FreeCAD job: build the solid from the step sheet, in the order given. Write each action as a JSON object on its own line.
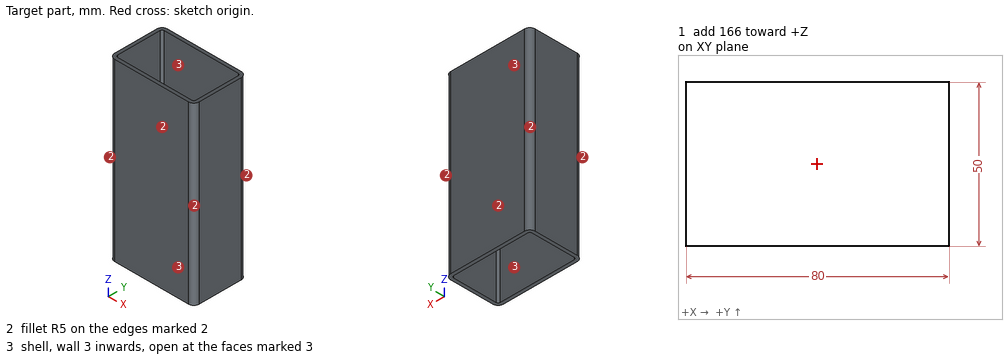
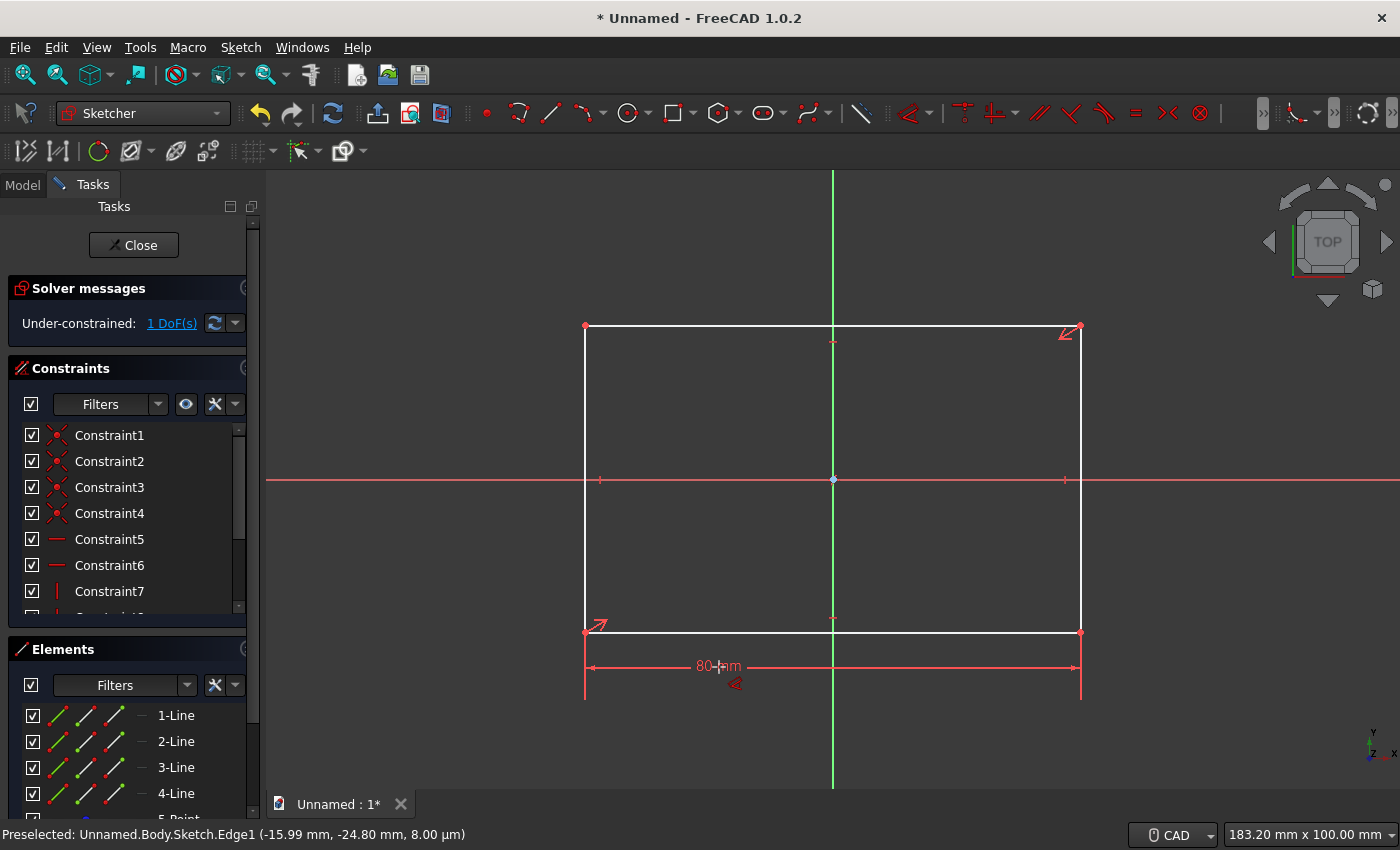
{"action": "left_click", "coordinate": [1081, 541]}
{"action": "left_click", "coordinate": [1115, 409]}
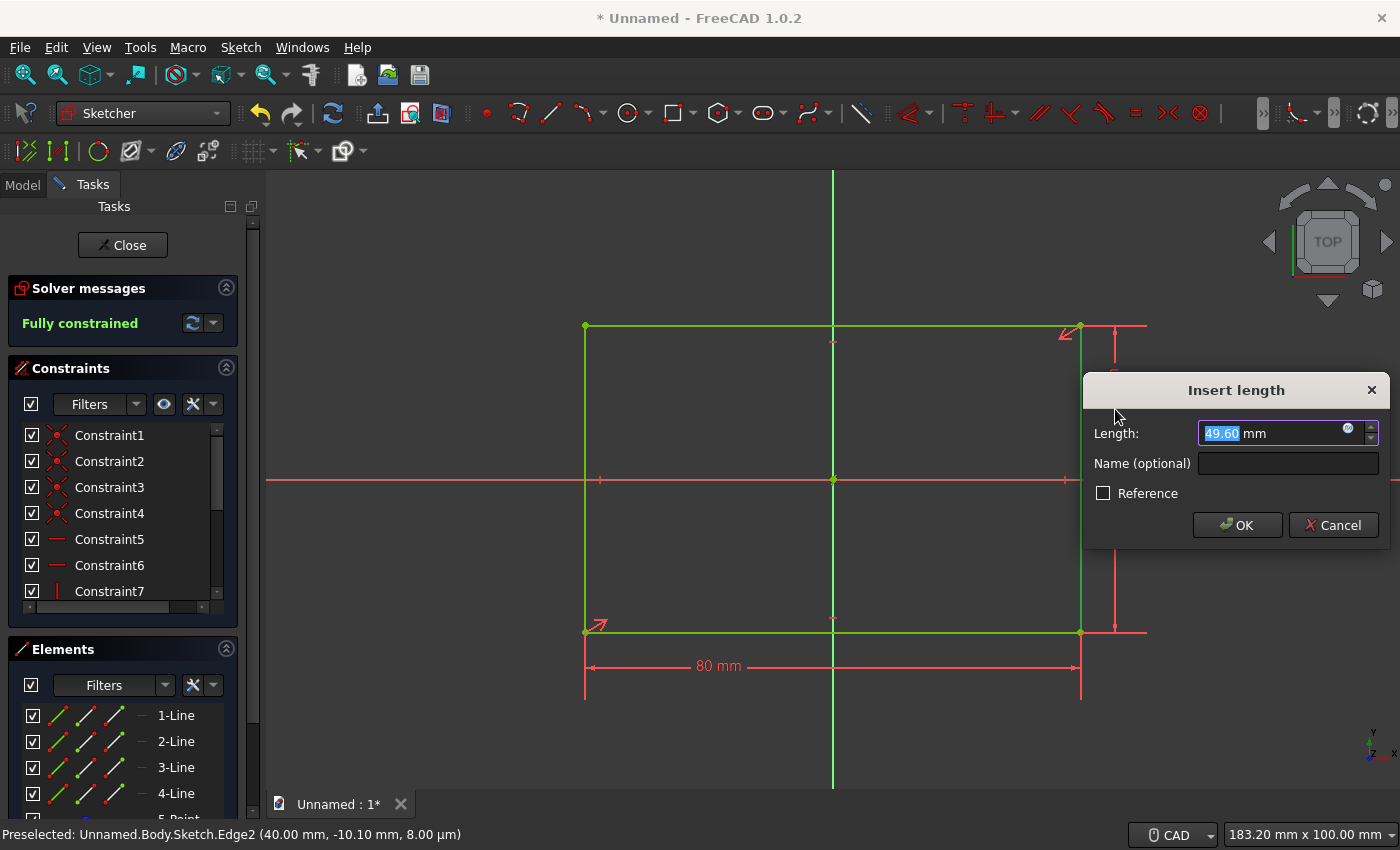
{"action": "type", "text": "50"}
{"action": "key", "text": "Return"}
{"action": "key", "text": "Escape"}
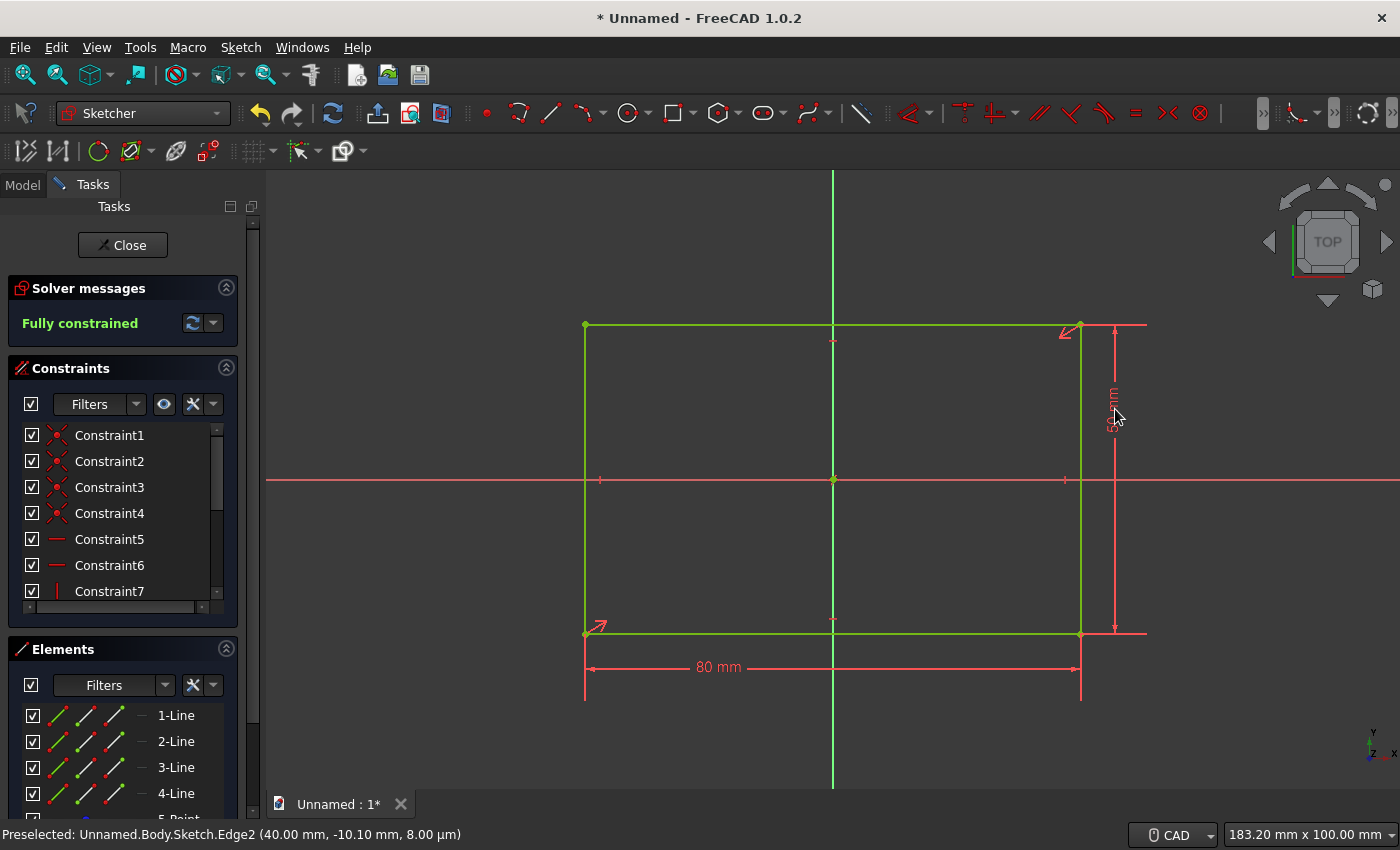
{"action": "left_click", "coordinate": [123, 245]}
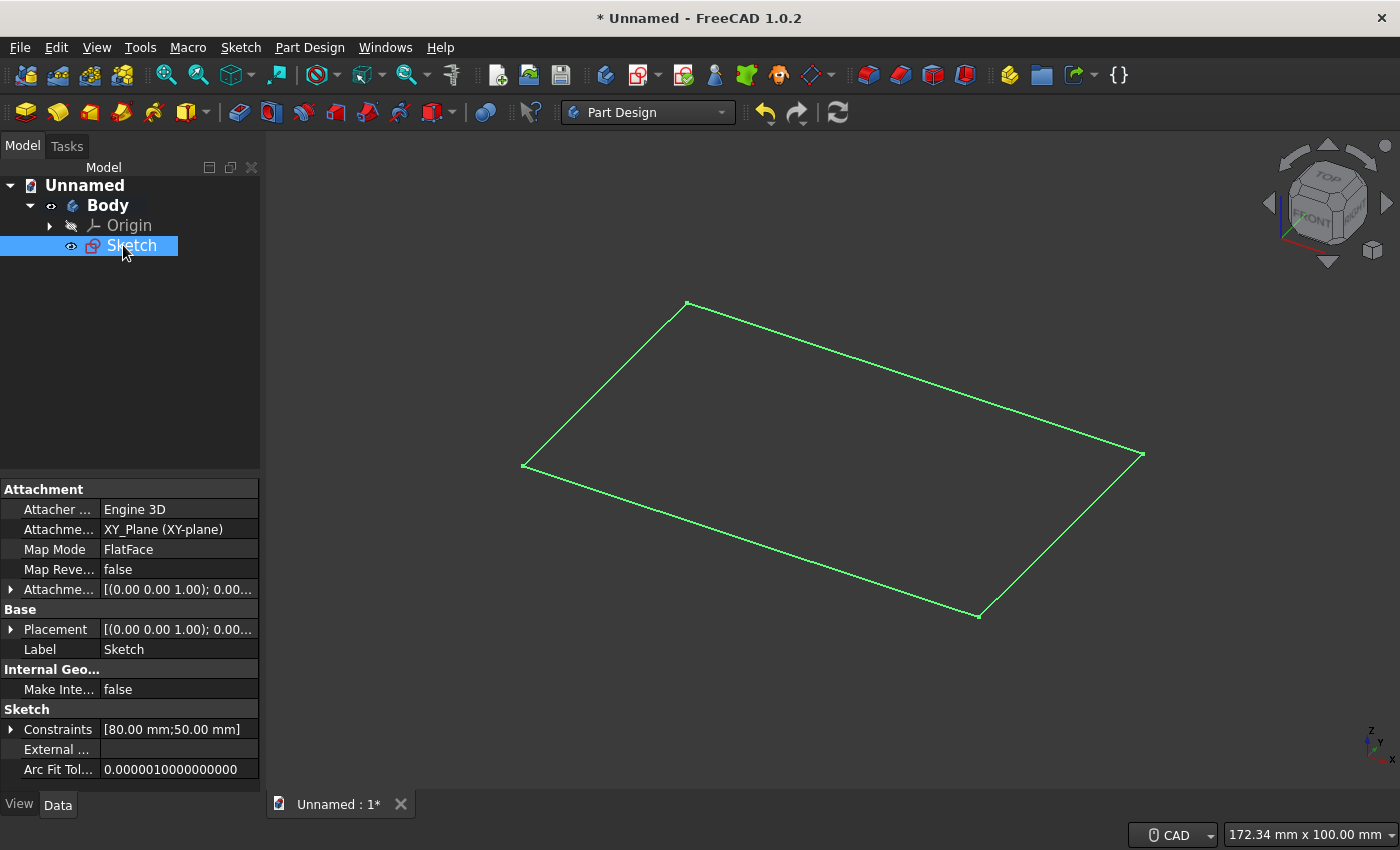
{"action": "left_click", "coordinate": [26, 112]}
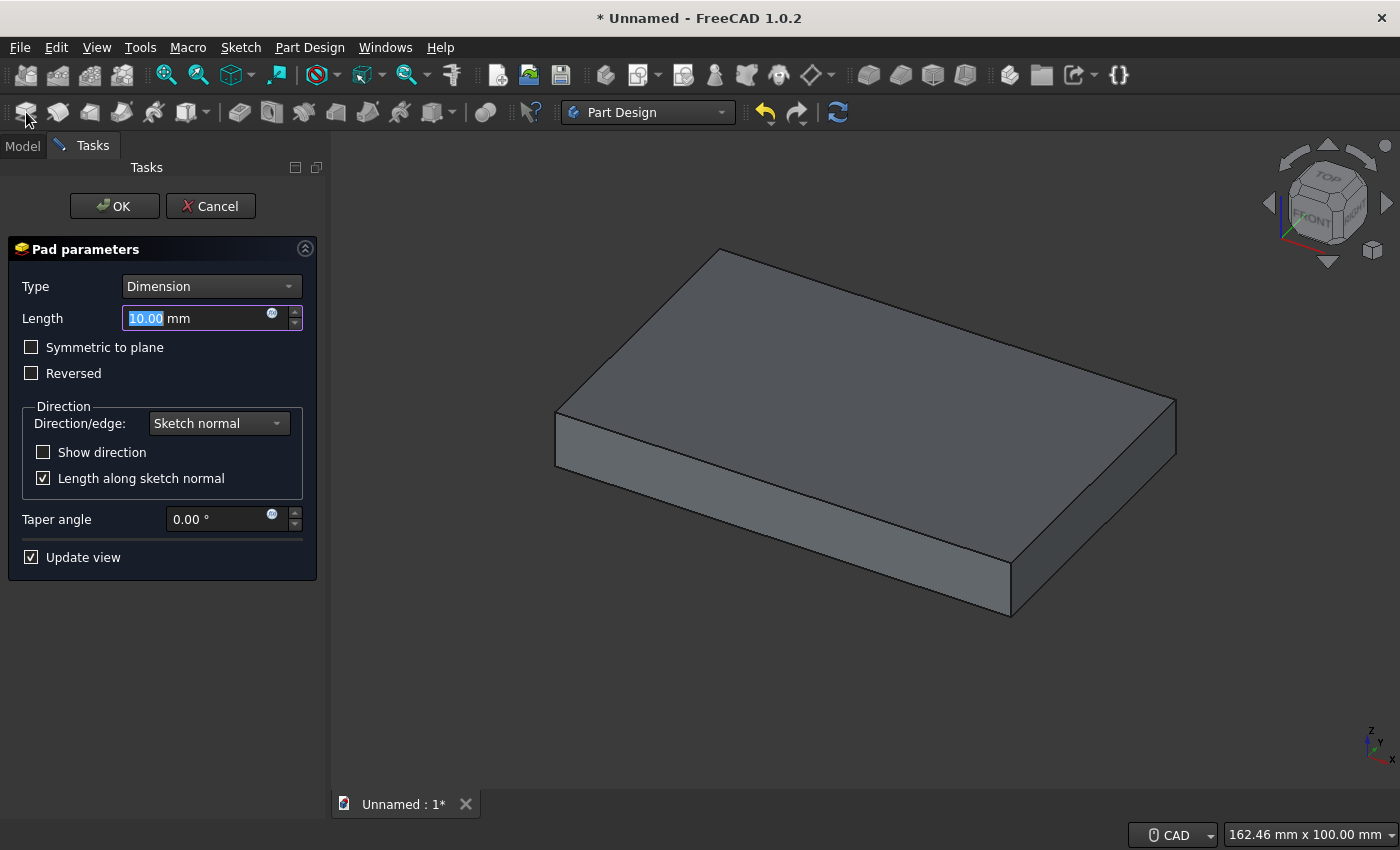
{"action": "type", "text": "166"}
{"action": "key", "text": "Tab"}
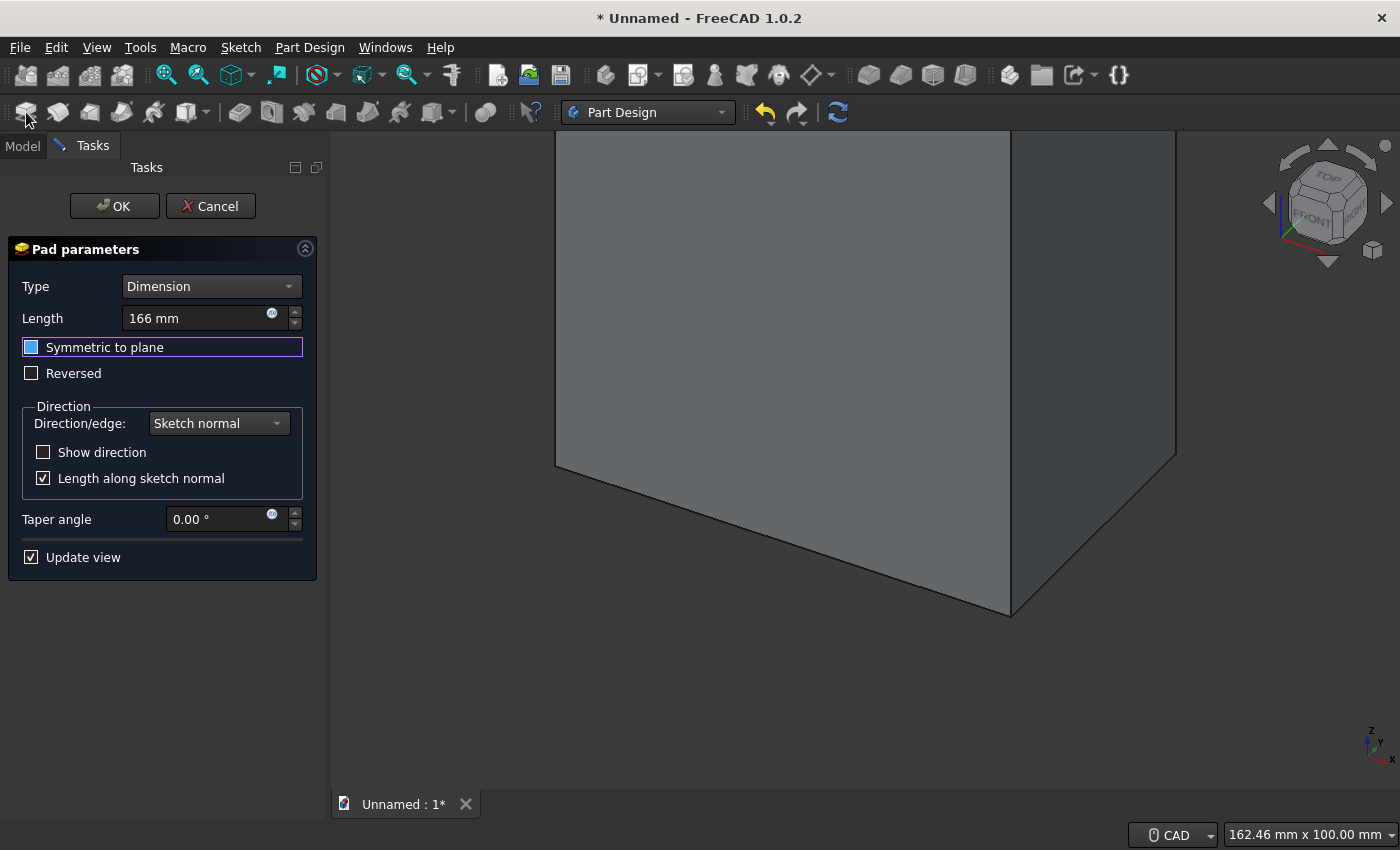
{"action": "left_click", "coordinate": [115, 206]}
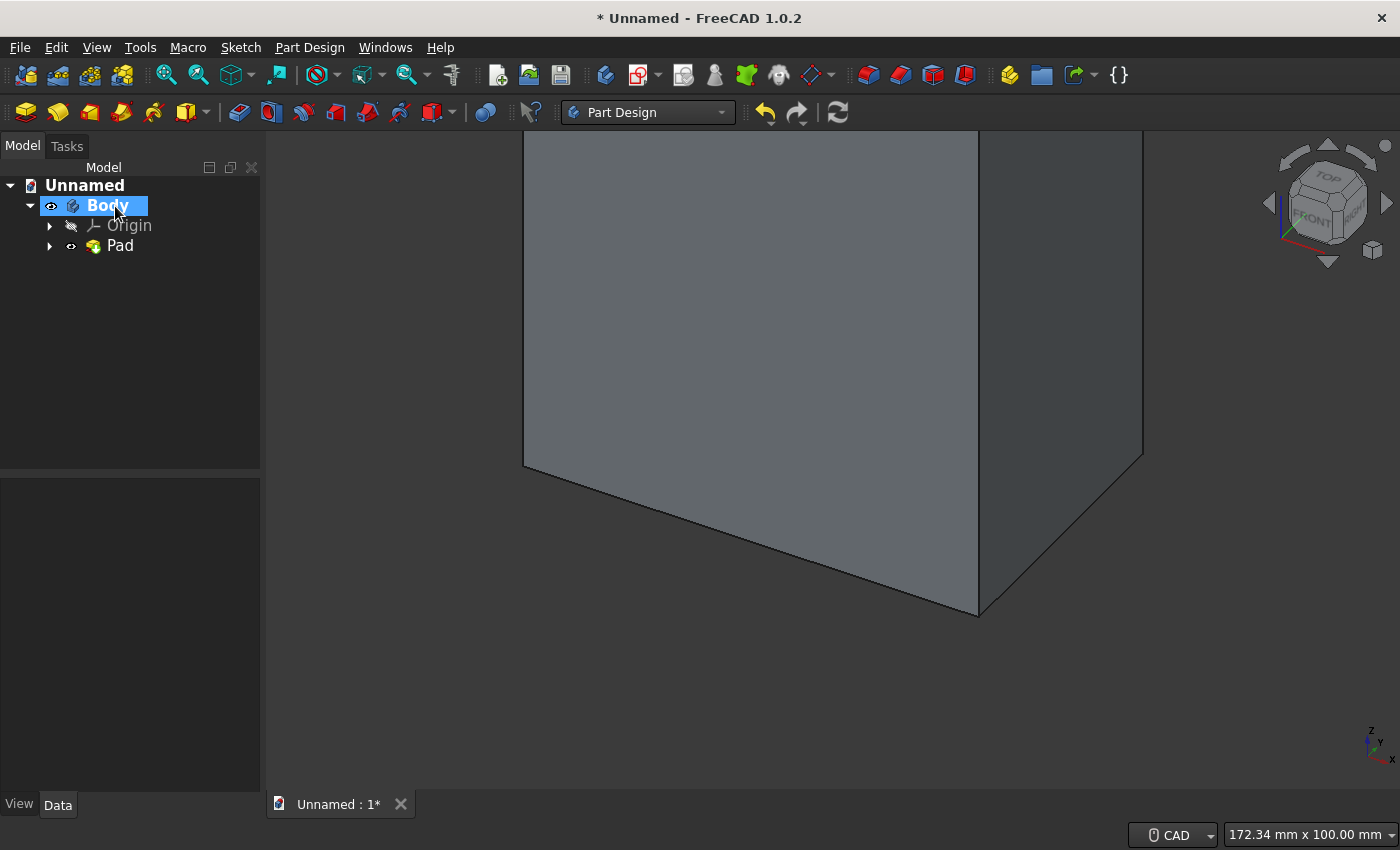
{"action": "key", "text": "v f"}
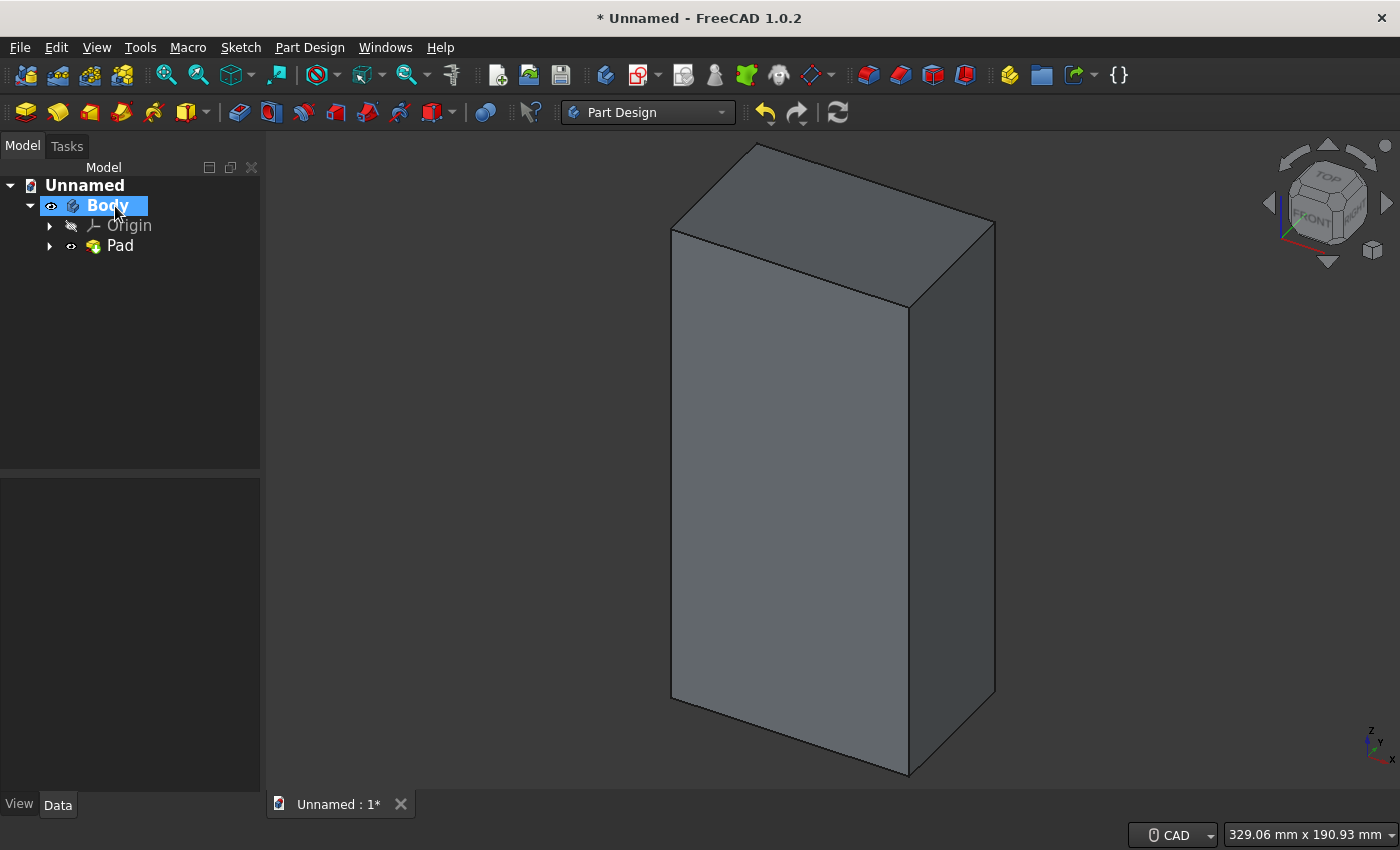
{"action": "left_click", "coordinate": [909, 541]}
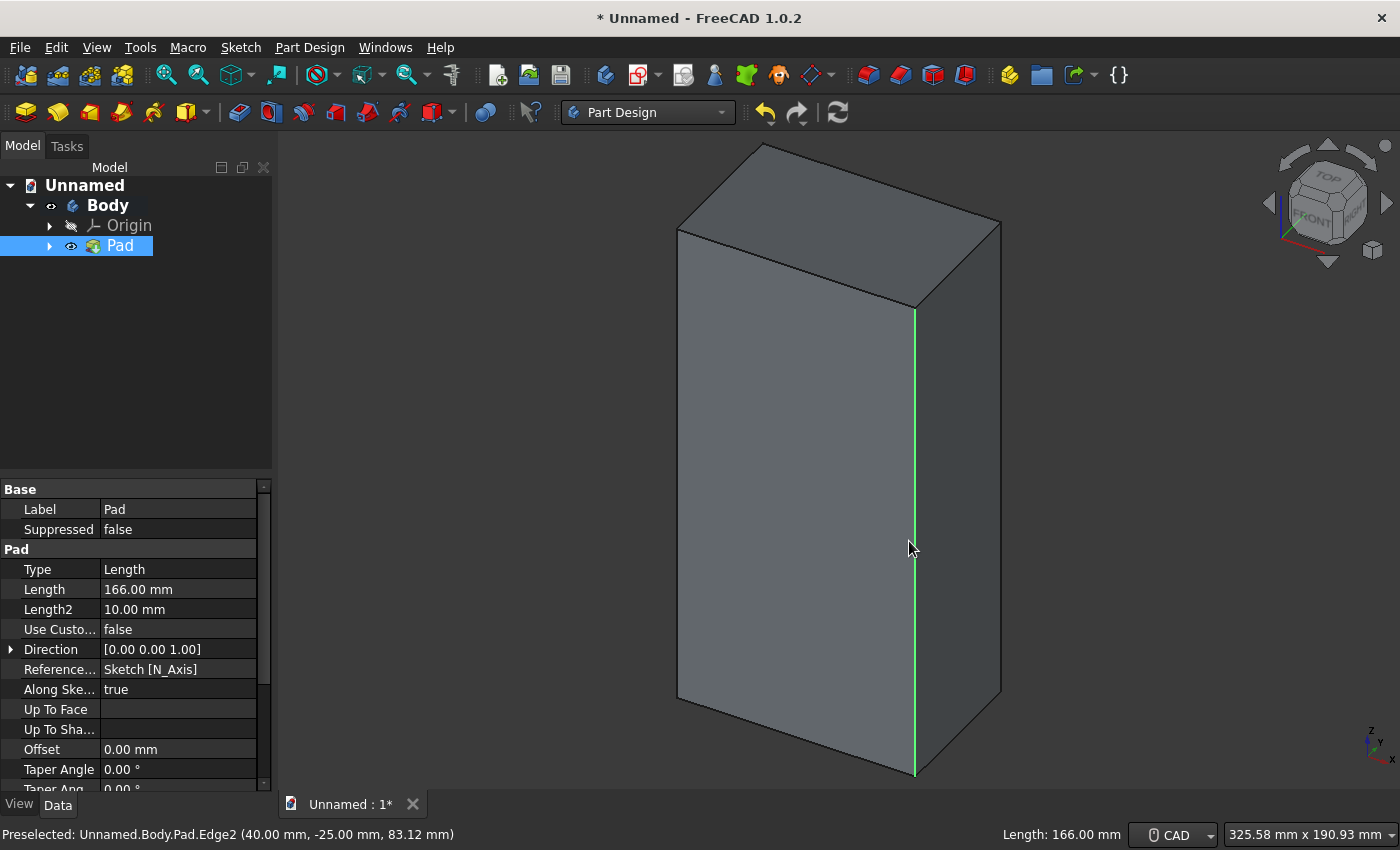
{"action": "key", "text": "0"}